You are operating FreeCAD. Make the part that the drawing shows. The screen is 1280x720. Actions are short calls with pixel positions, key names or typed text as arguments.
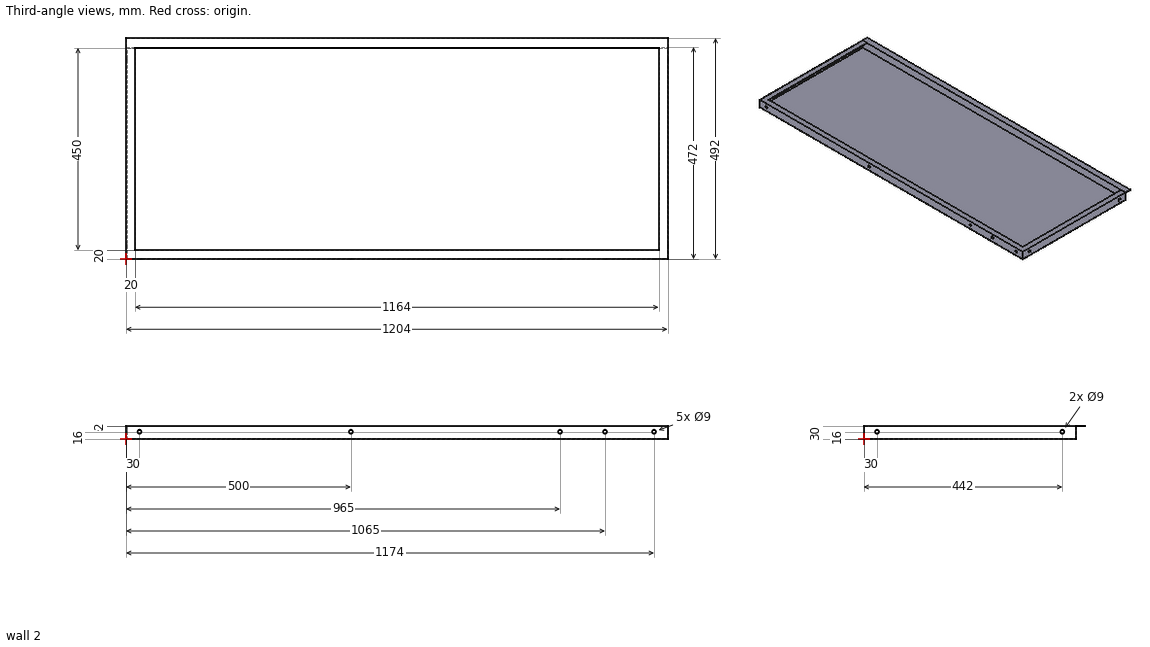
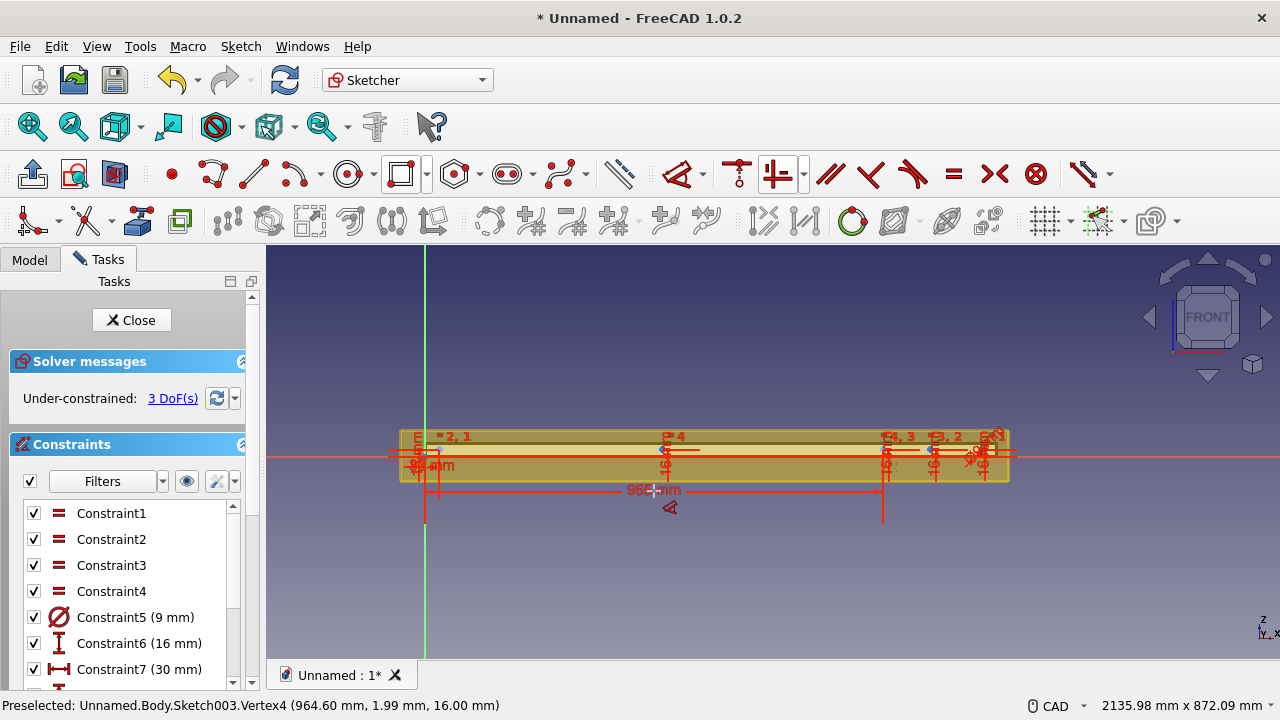
click(662, 450)
click(544, 491)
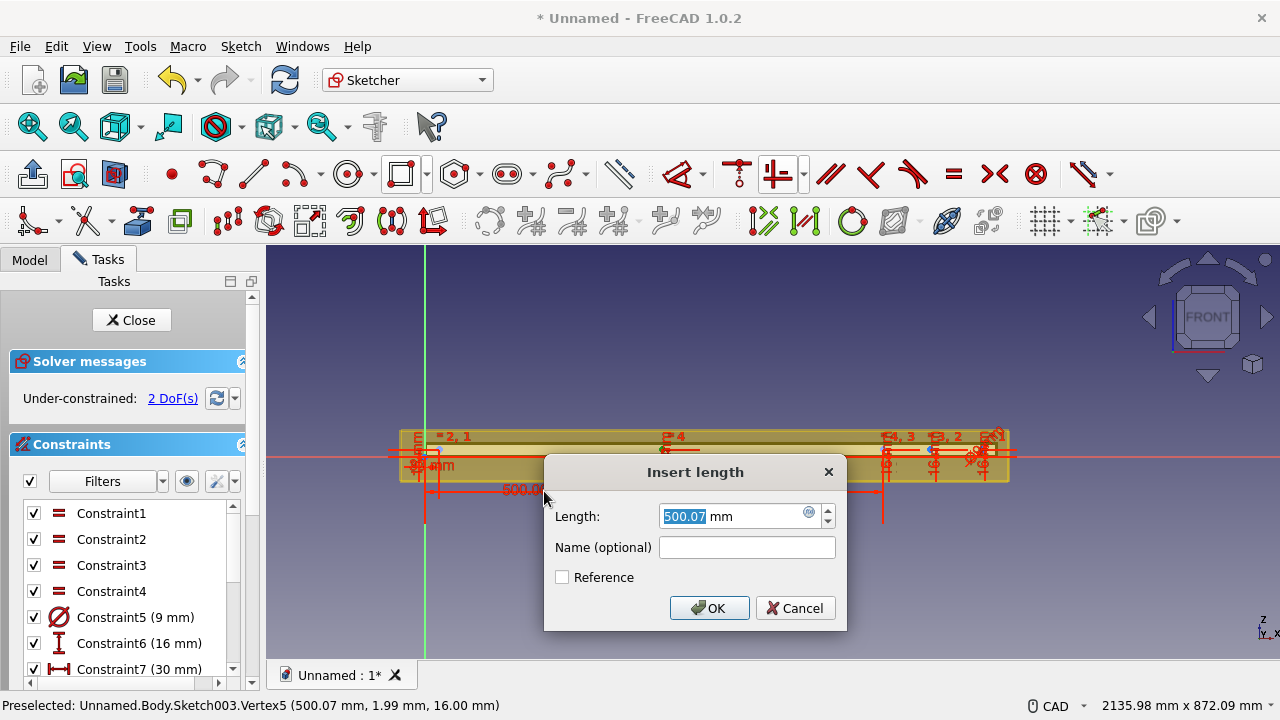
text(500)
key(Return)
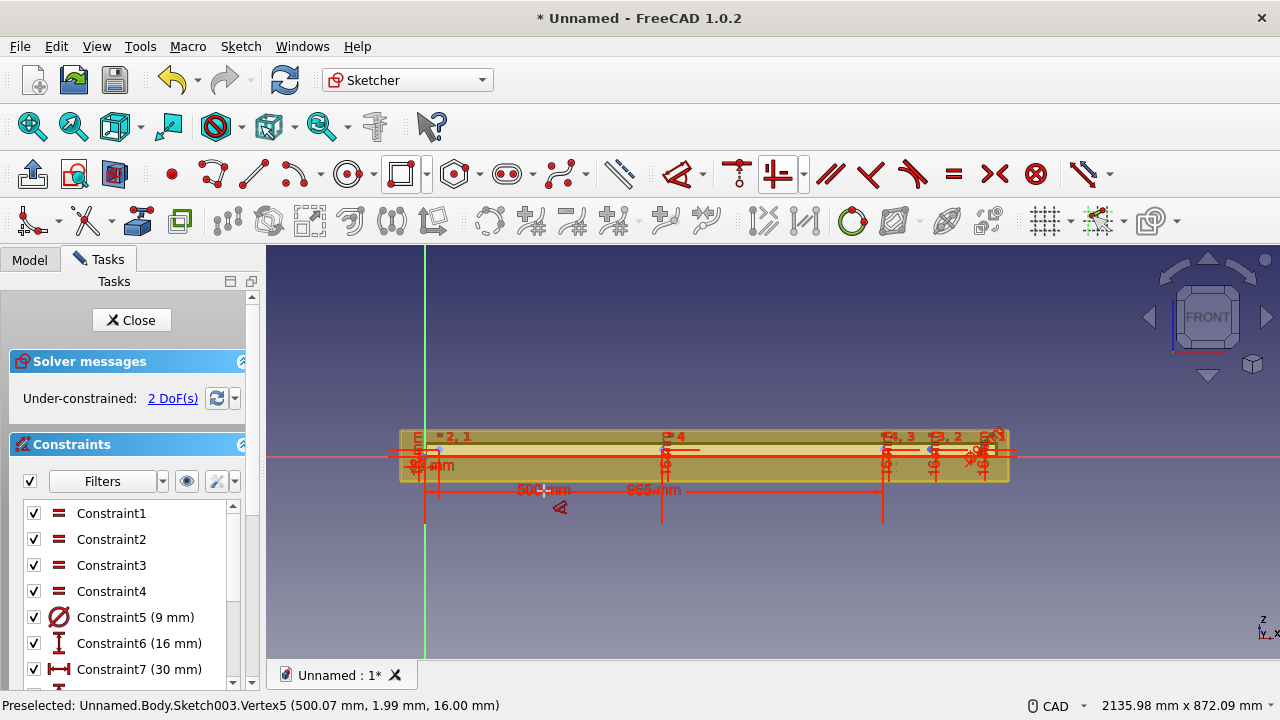
click(982, 450)
click(832, 491)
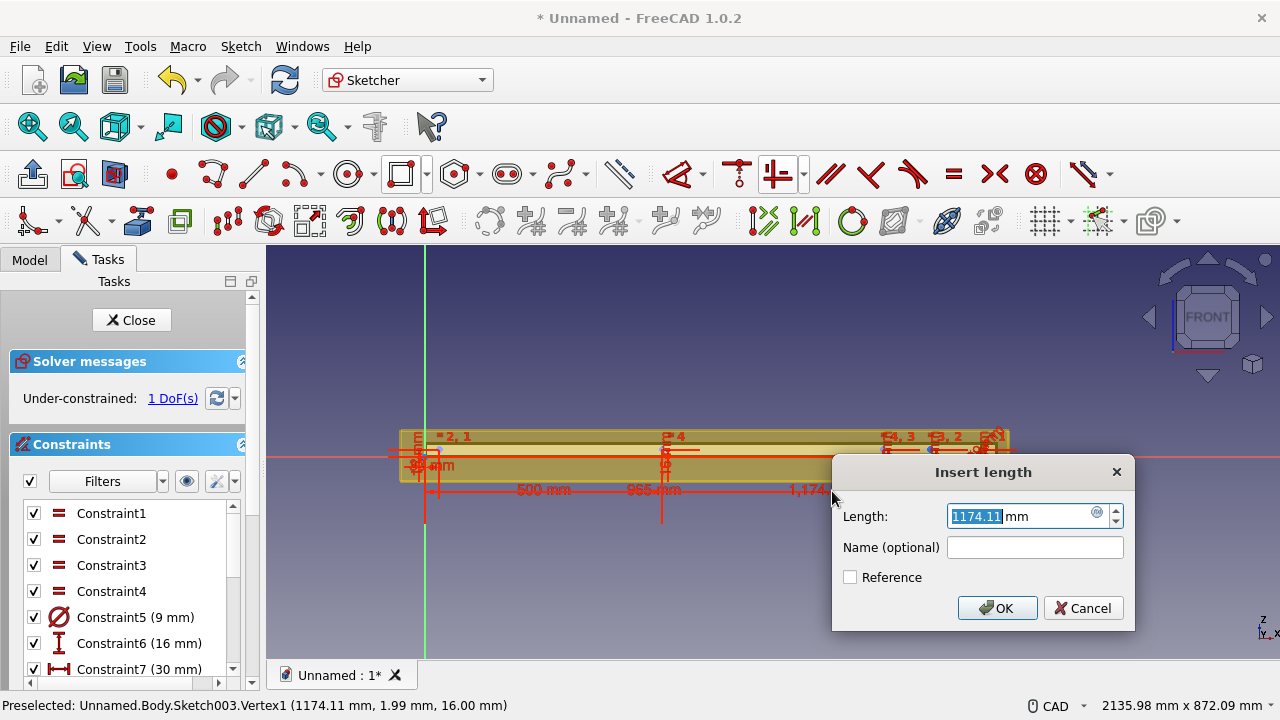
text(1174)
key(Return)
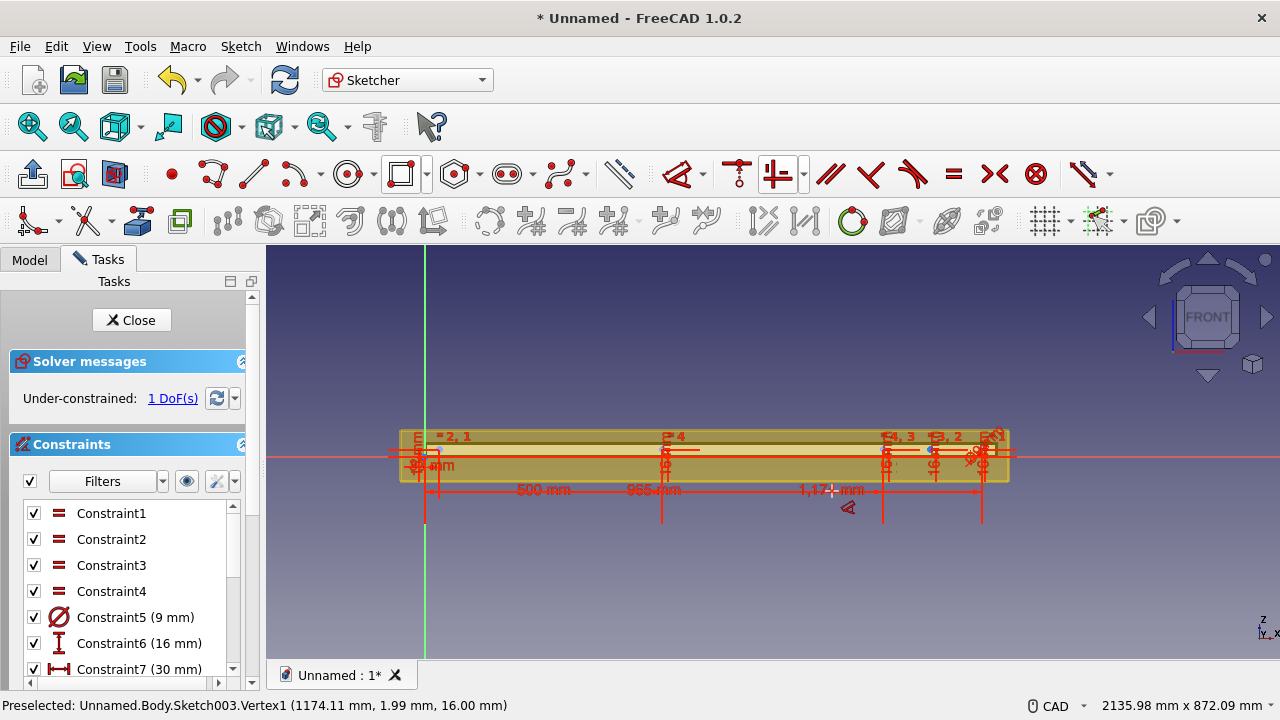
click(931, 450)
click(678, 416)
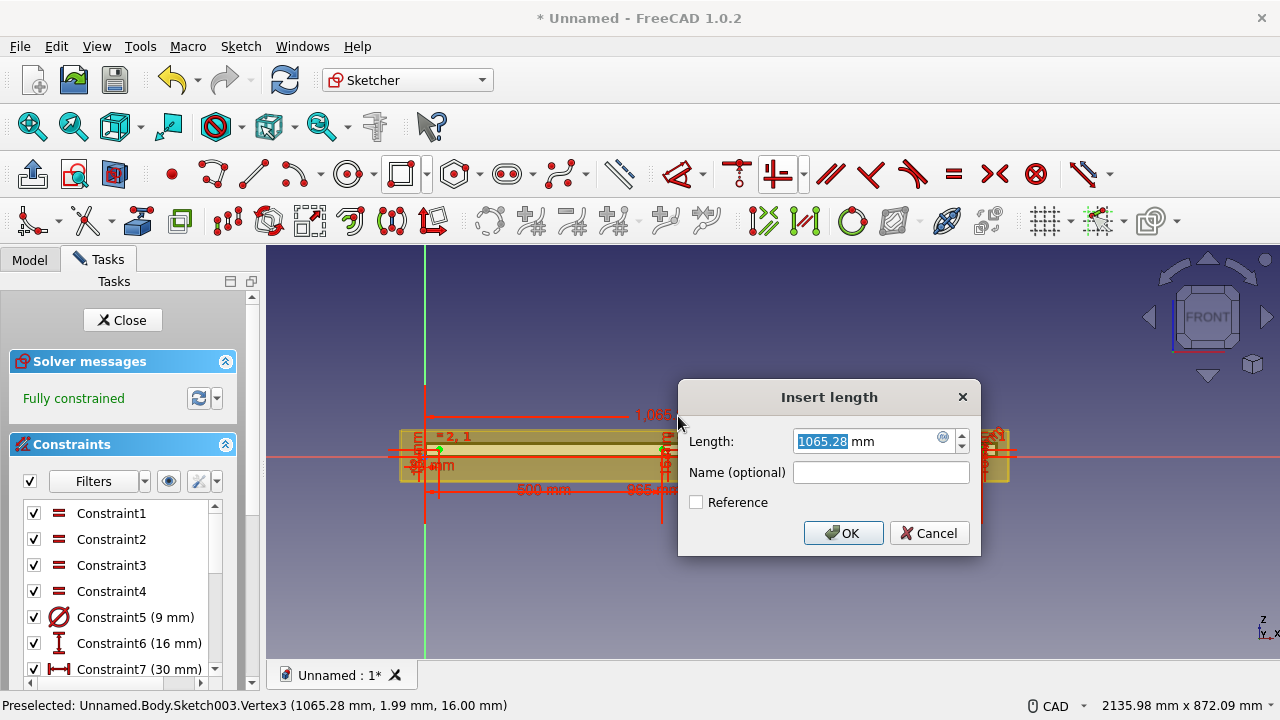
text(1065)
key(Return)
key(Escape)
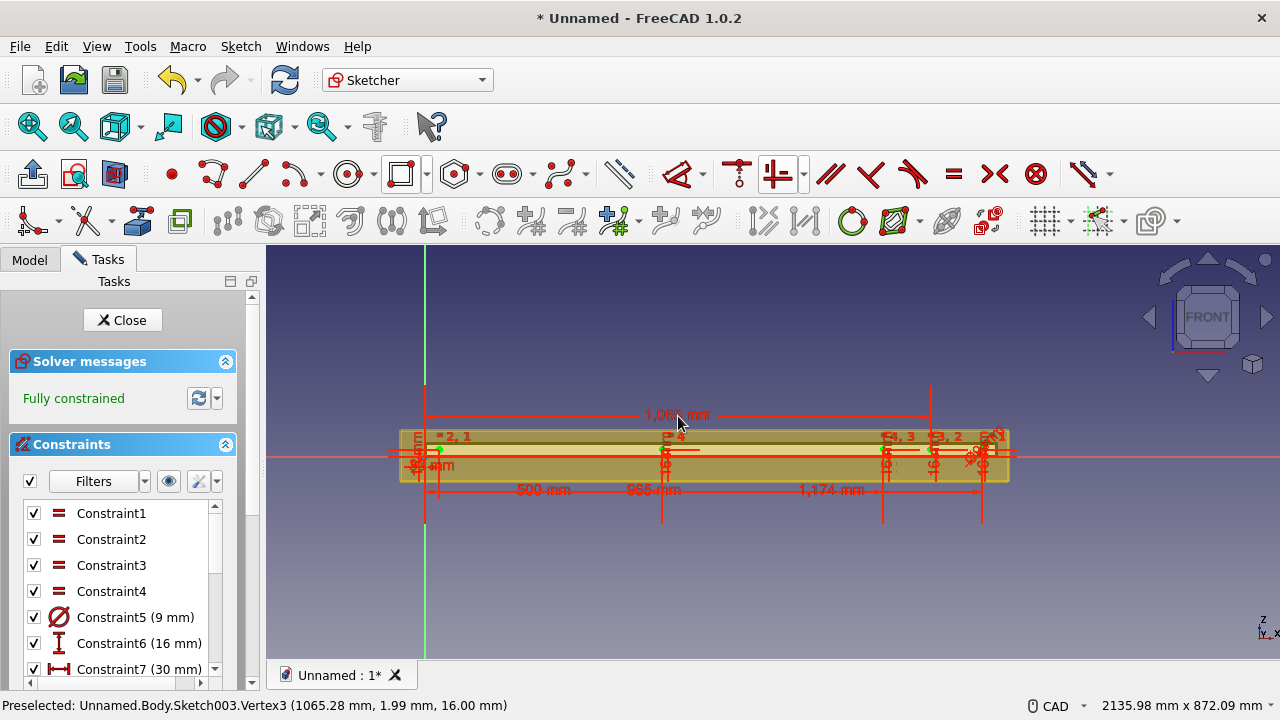
click(123, 320)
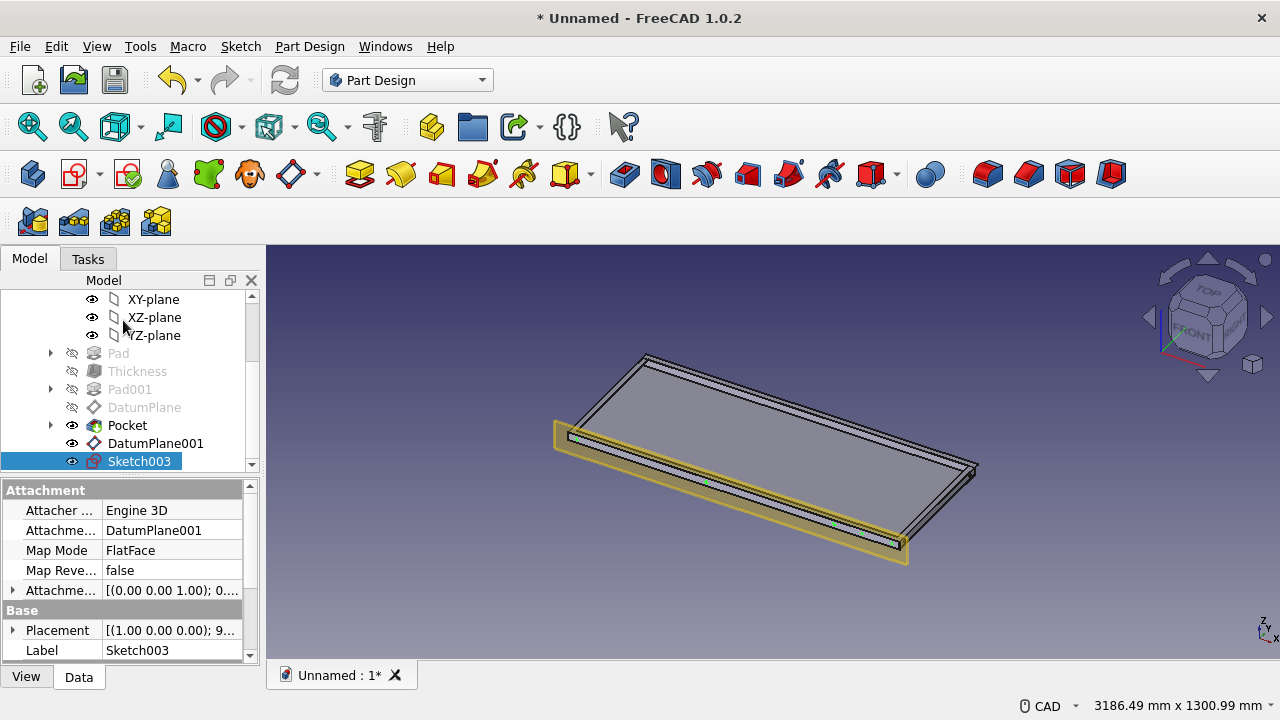
click(625, 174)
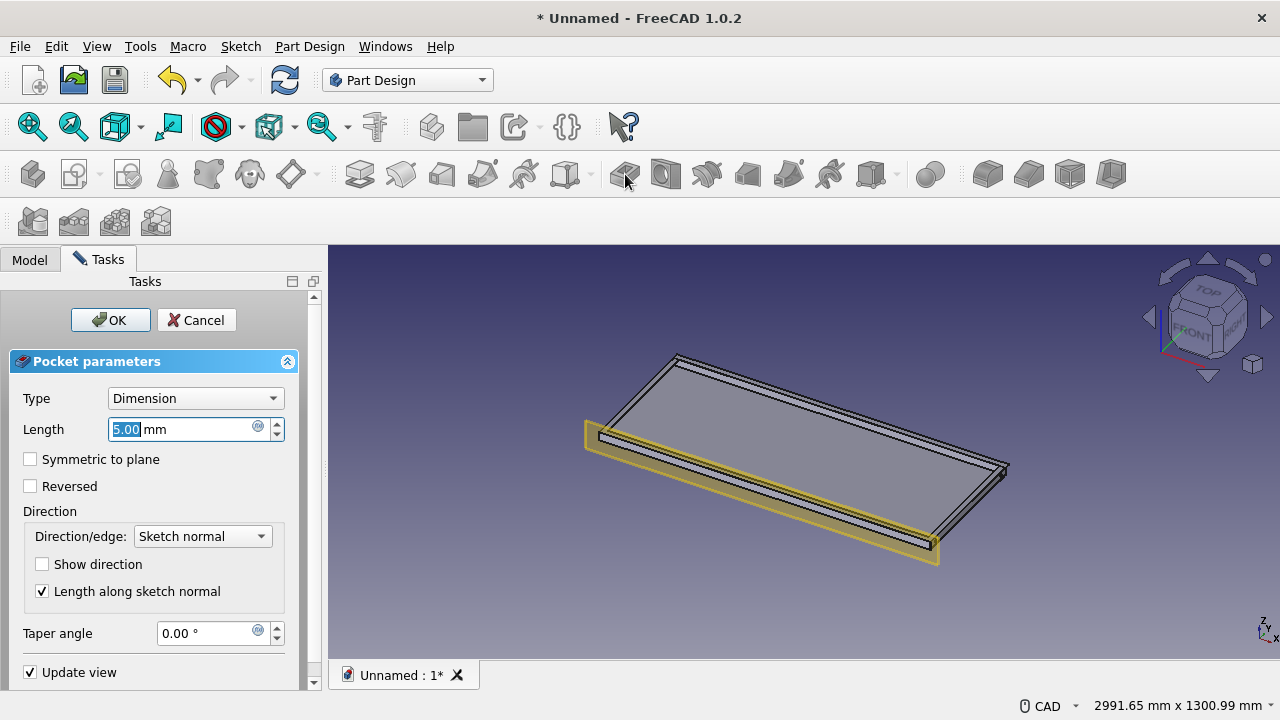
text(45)
key(Tab)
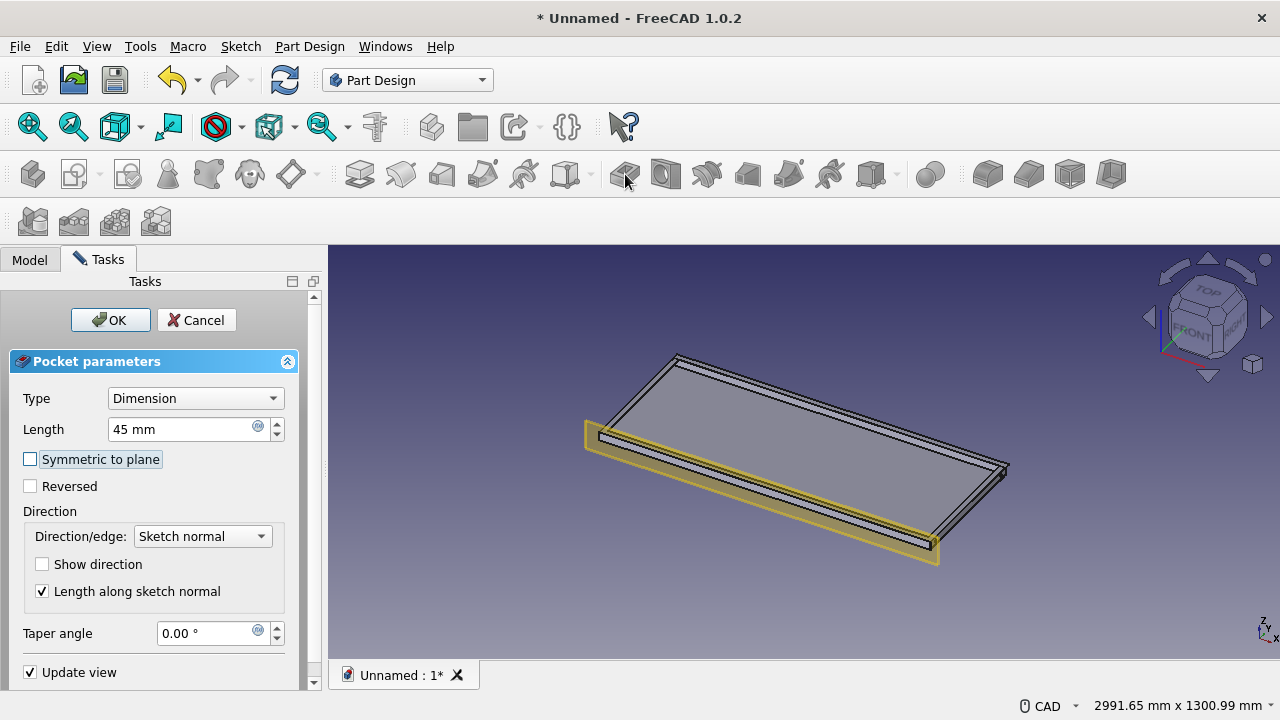
click(31, 486)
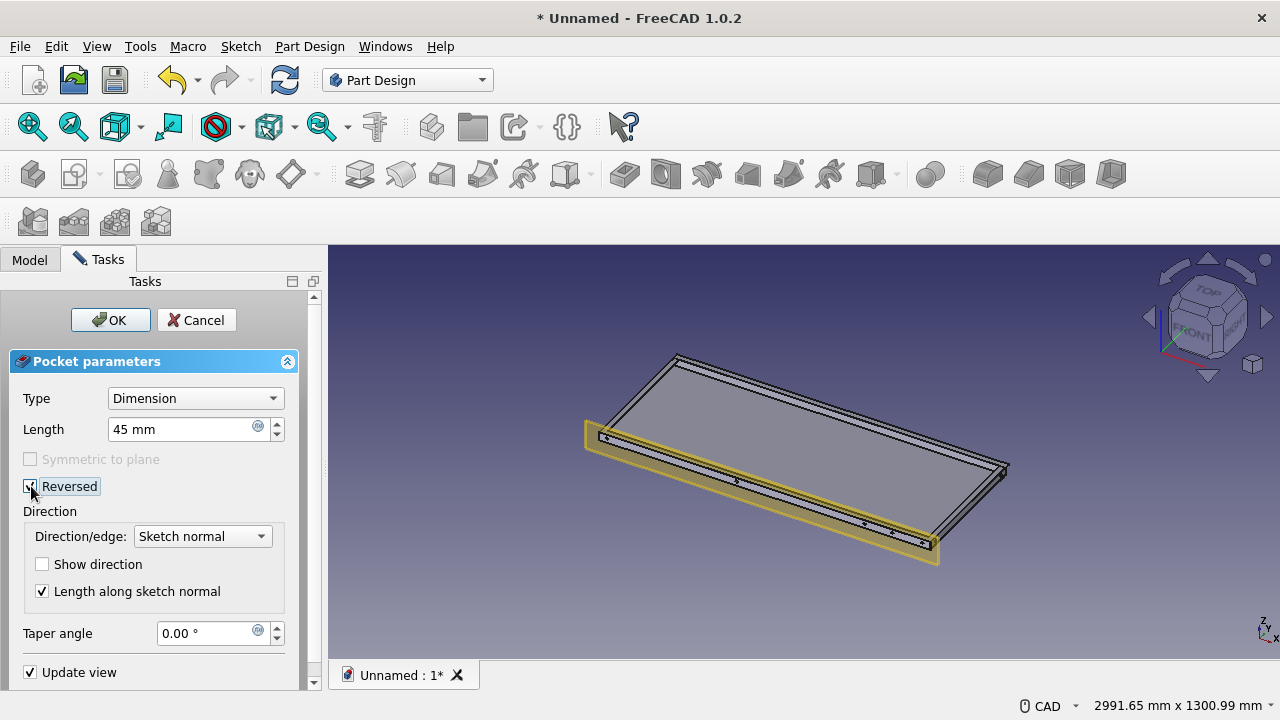
click(111, 320)